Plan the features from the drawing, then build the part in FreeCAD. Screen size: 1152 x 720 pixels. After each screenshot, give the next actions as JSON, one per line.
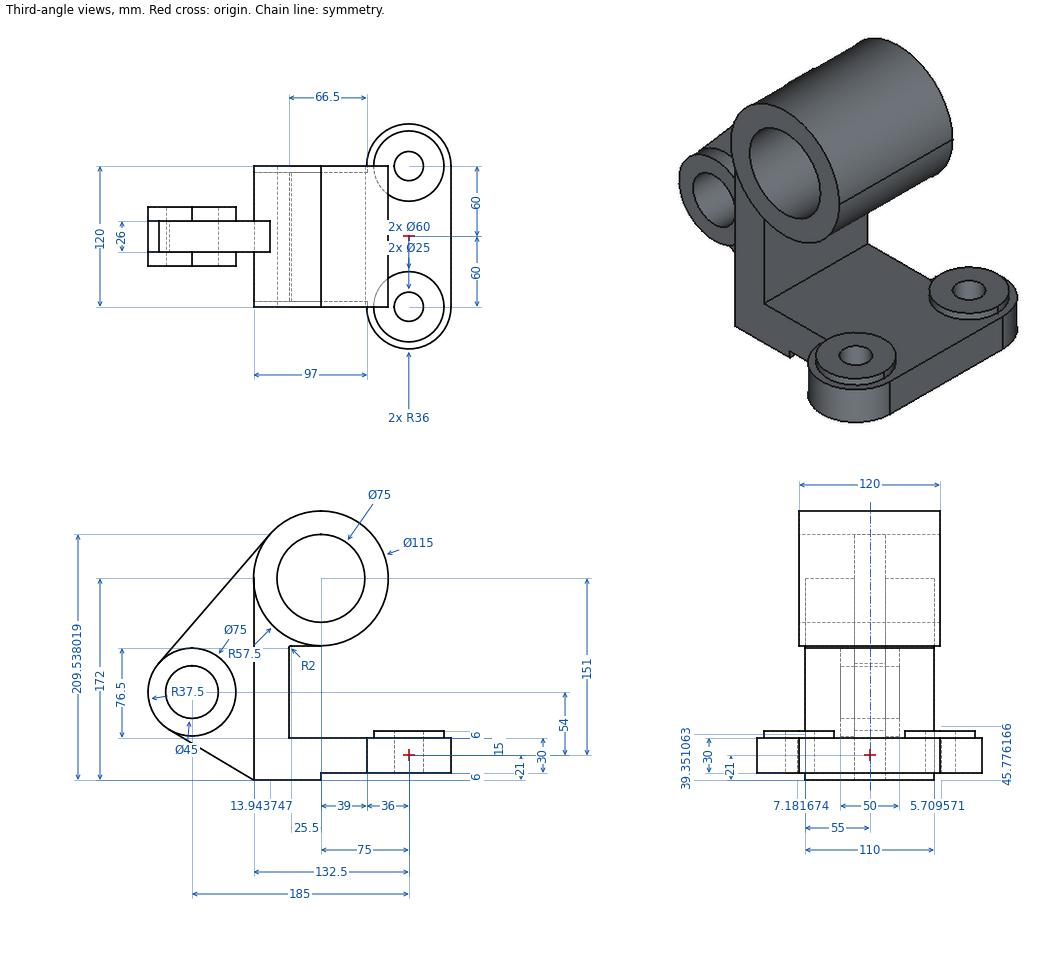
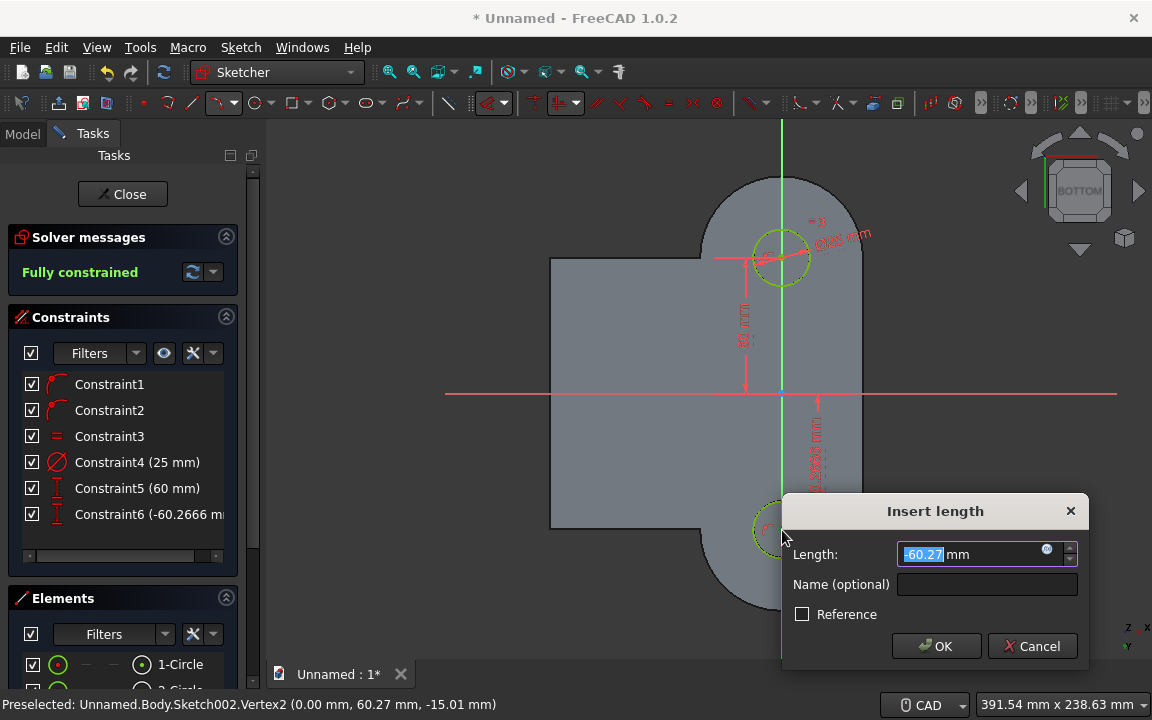
{"action": "type", "text": "-60"}
{"action": "key", "text": "Return"}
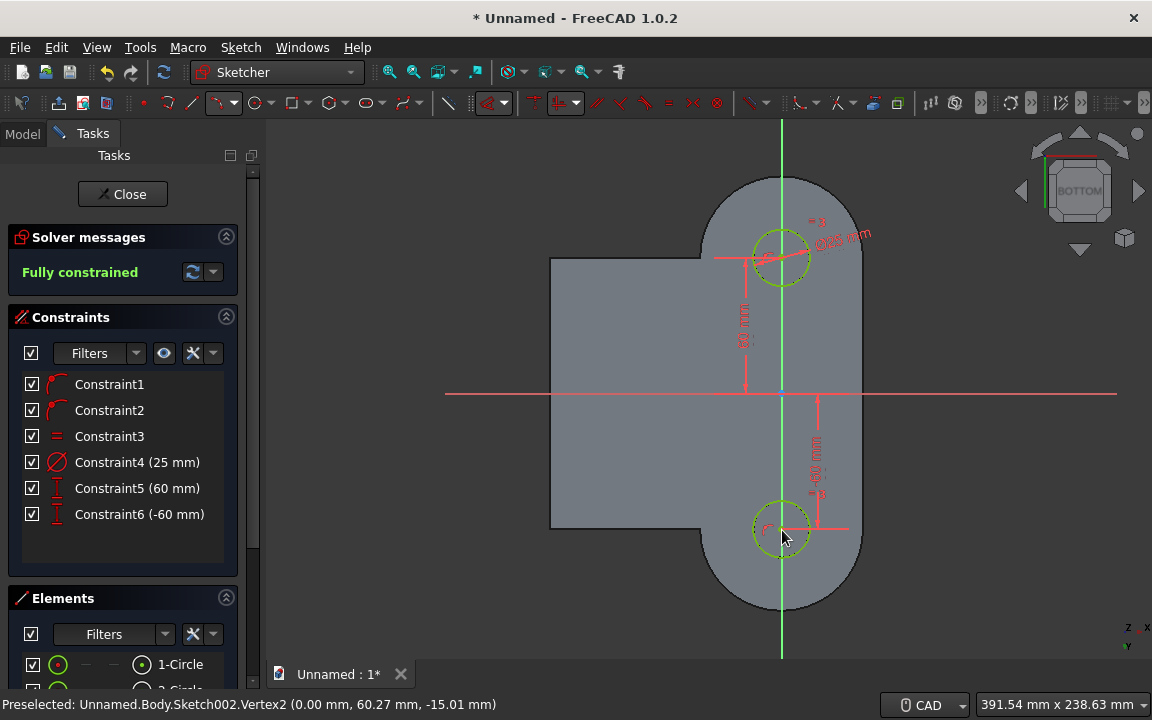
{"action": "left_click", "coordinate": [123, 194]}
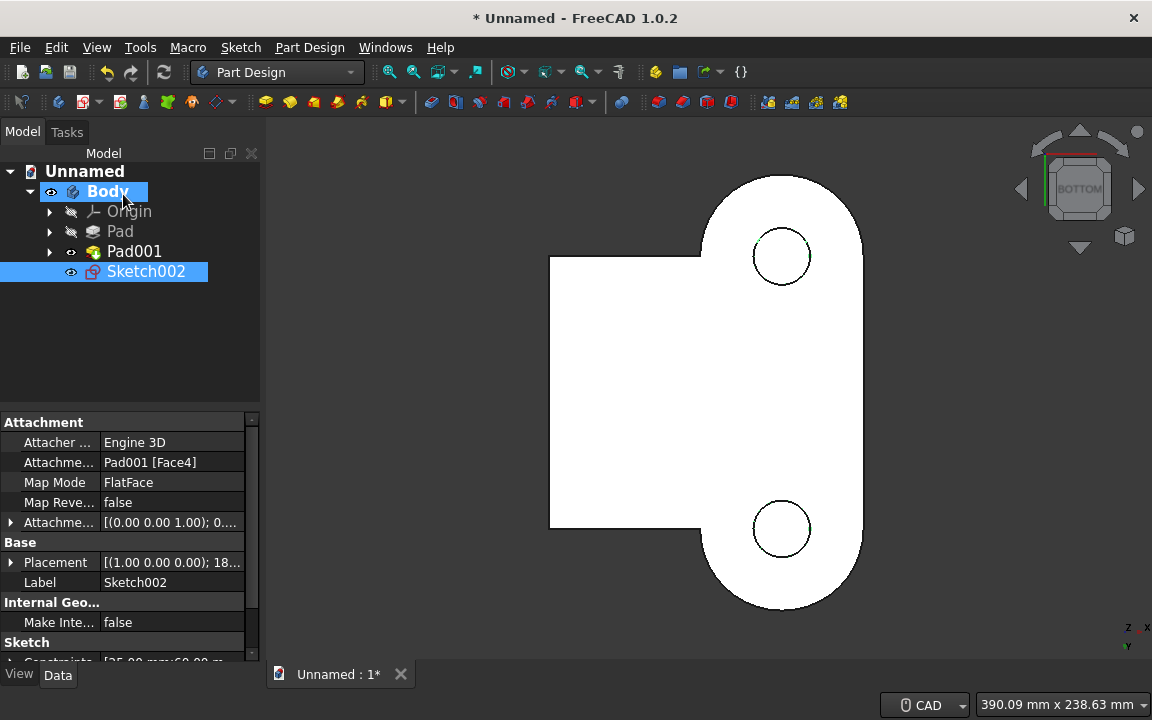
{"action": "left_click", "coordinate": [432, 102]}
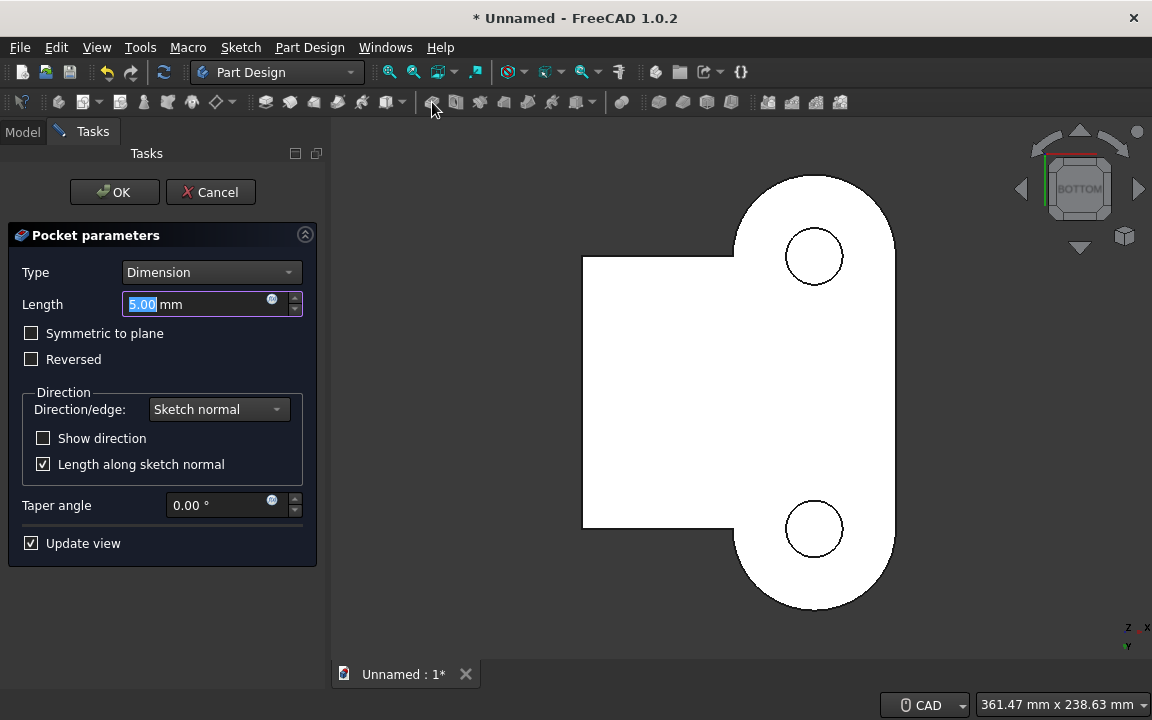
{"action": "left_click", "coordinate": [212, 272]}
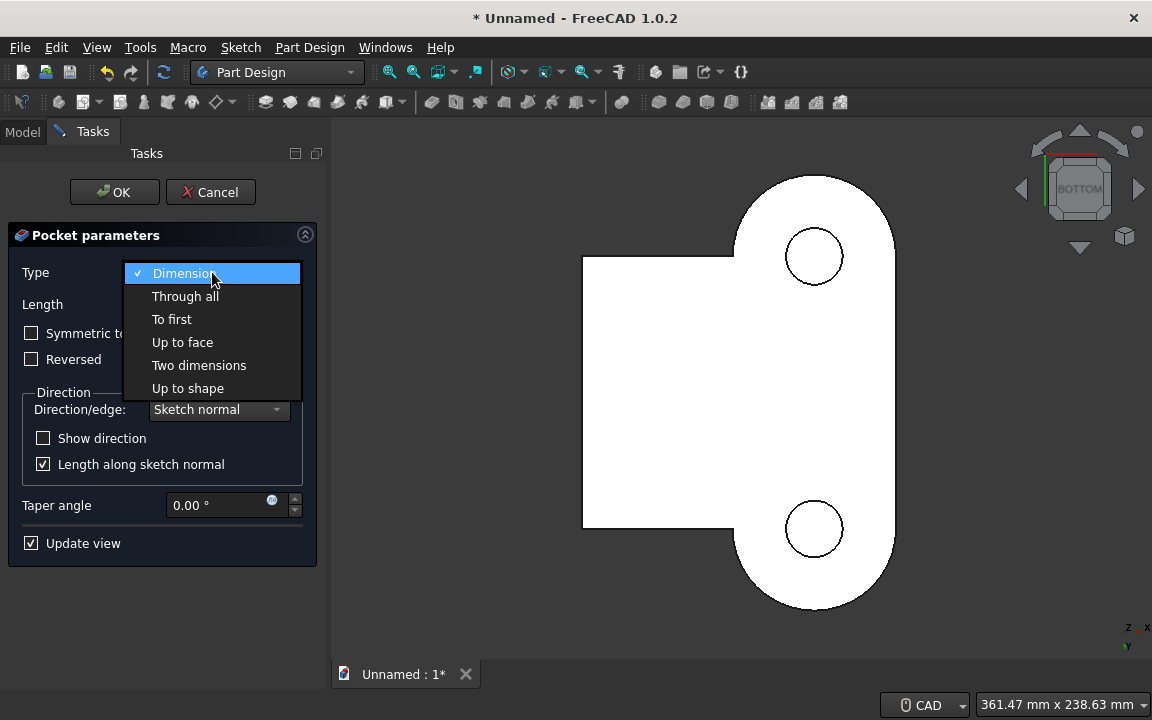
{"action": "left_click", "coordinate": [212, 296]}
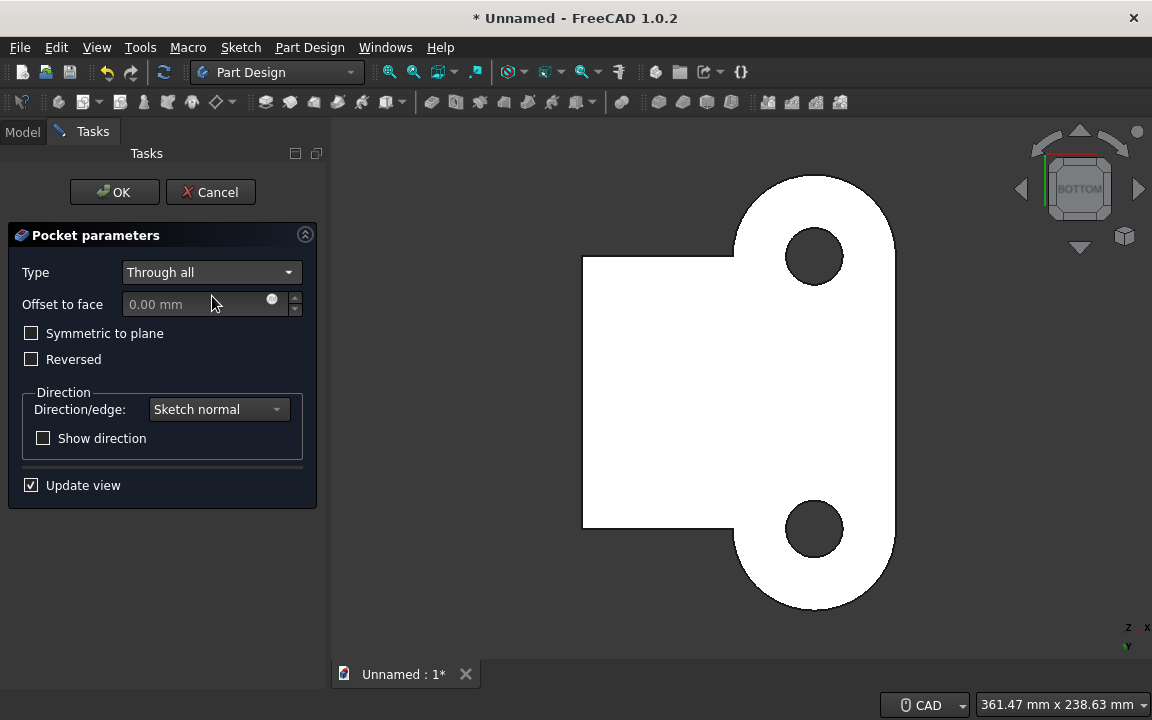
{"action": "left_click", "coordinate": [115, 192]}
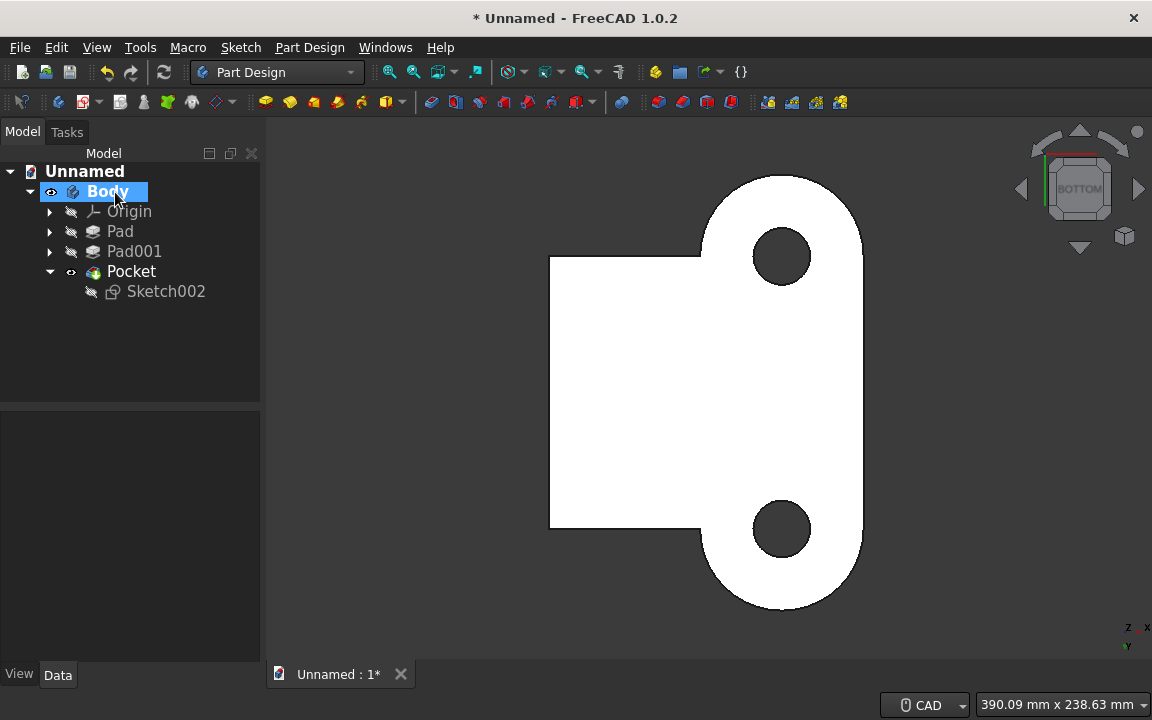
{"action": "left_click", "coordinate": [60, 102]}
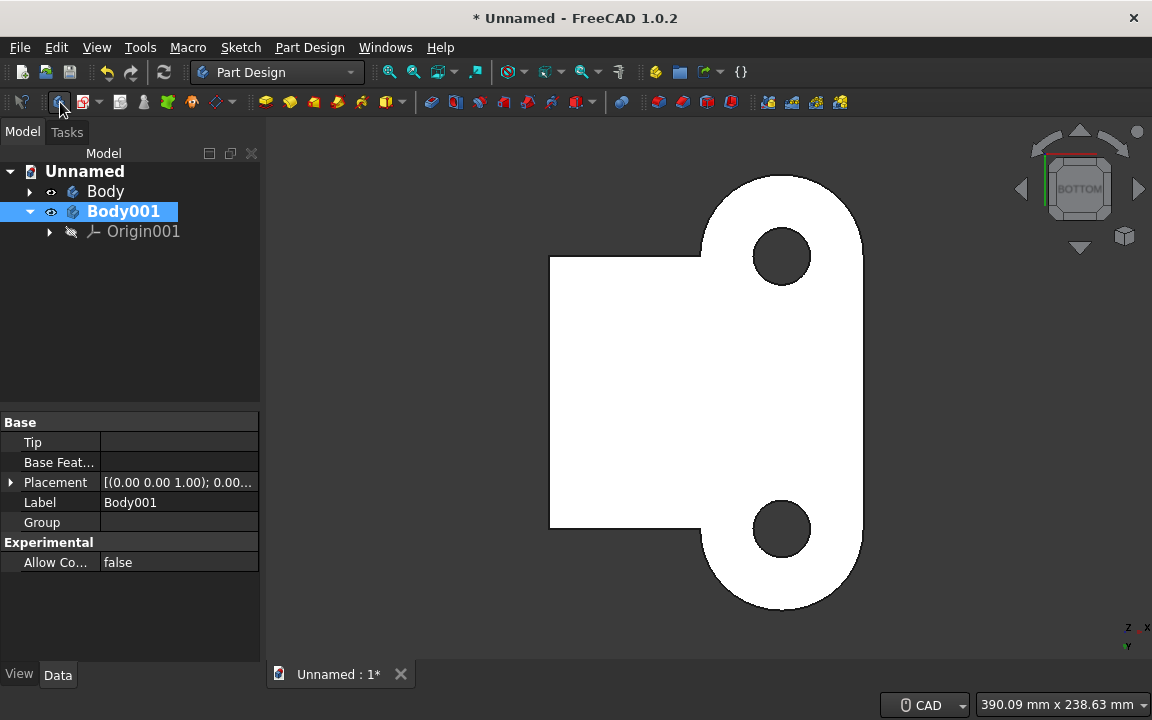
{"action": "left_click", "coordinate": [306, 619]}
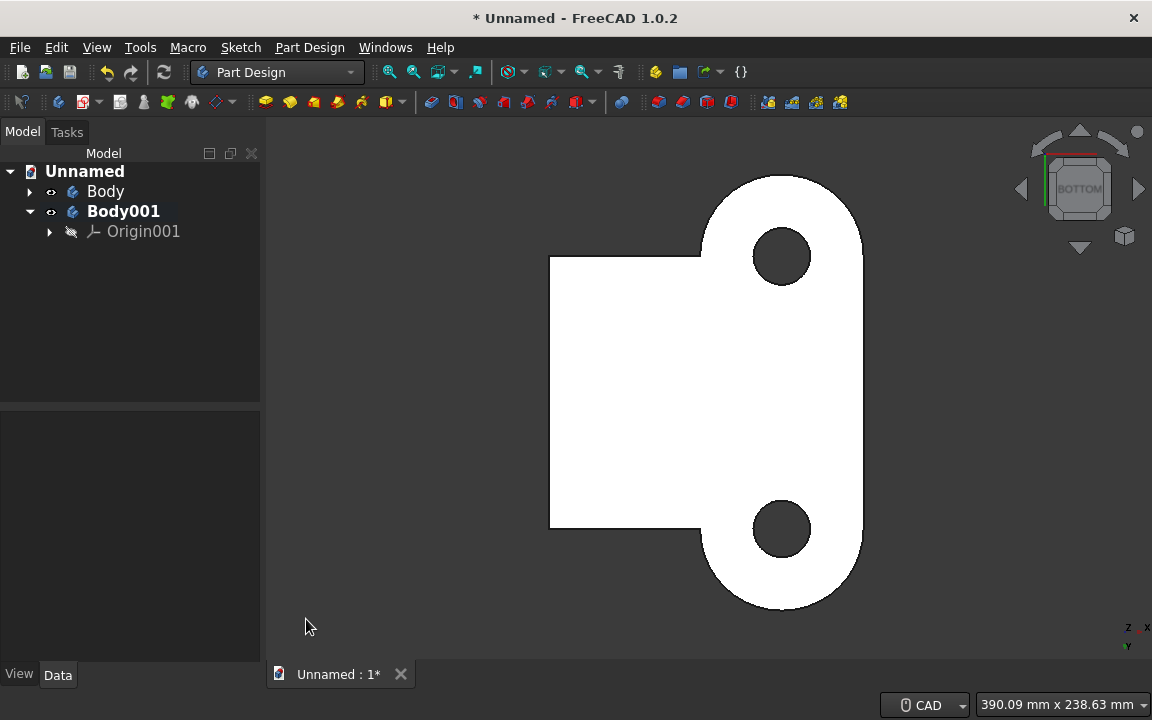
{"action": "left_click", "coordinate": [84, 102]}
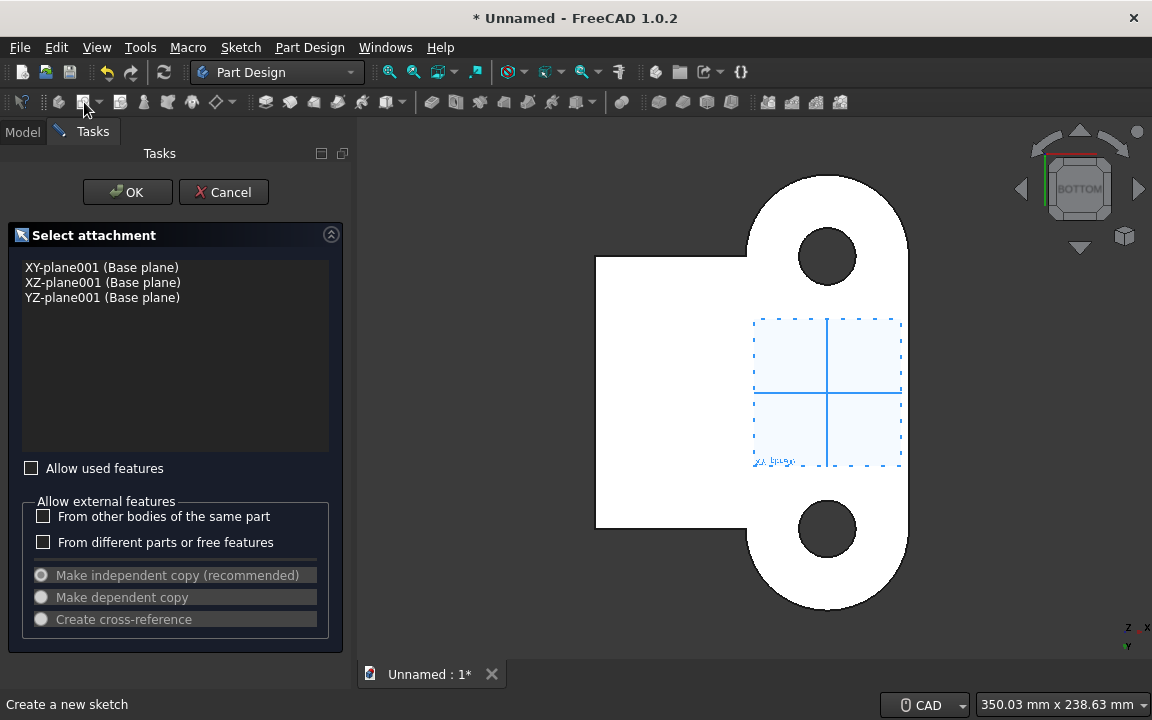
{"action": "left_click", "coordinate": [82, 282]}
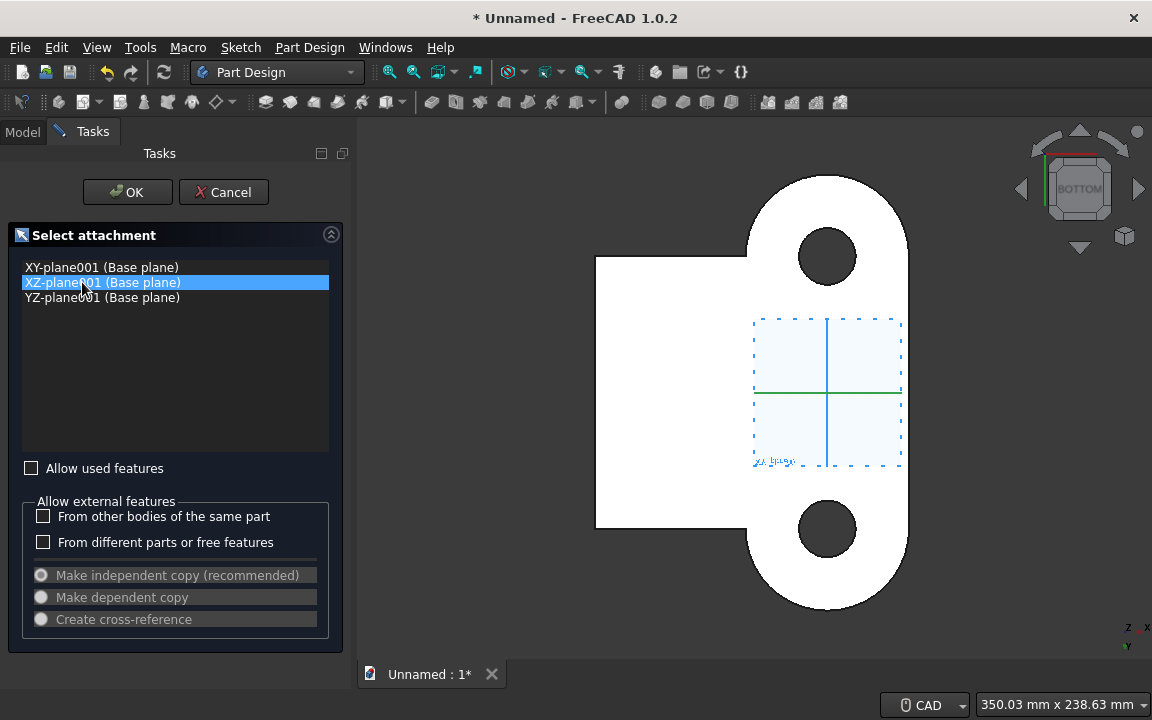
{"action": "left_click", "coordinate": [128, 192]}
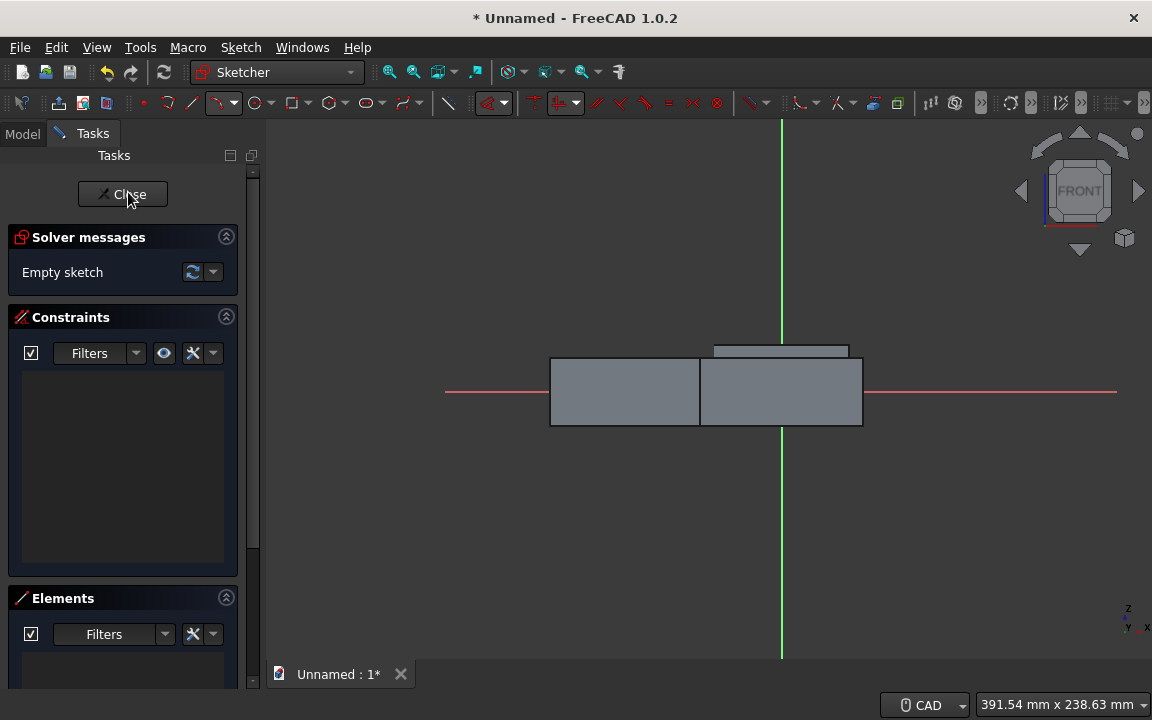
{"action": "scroll", "coordinate": [651, 631], "scroll_direction": "down", "scroll_amount": 3}